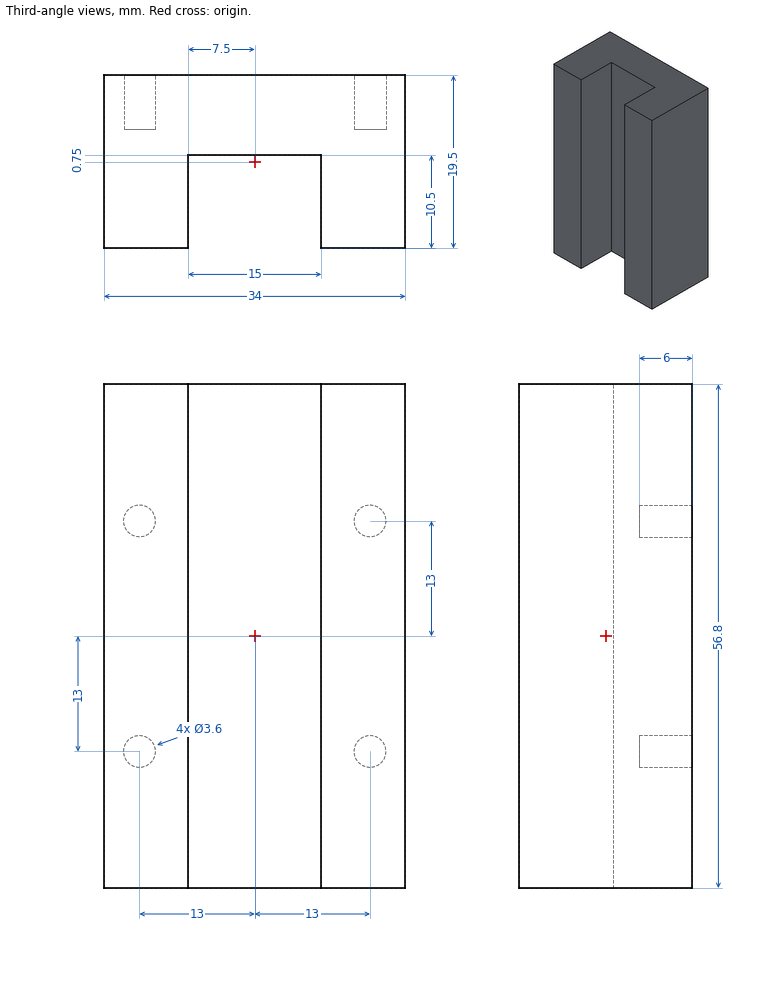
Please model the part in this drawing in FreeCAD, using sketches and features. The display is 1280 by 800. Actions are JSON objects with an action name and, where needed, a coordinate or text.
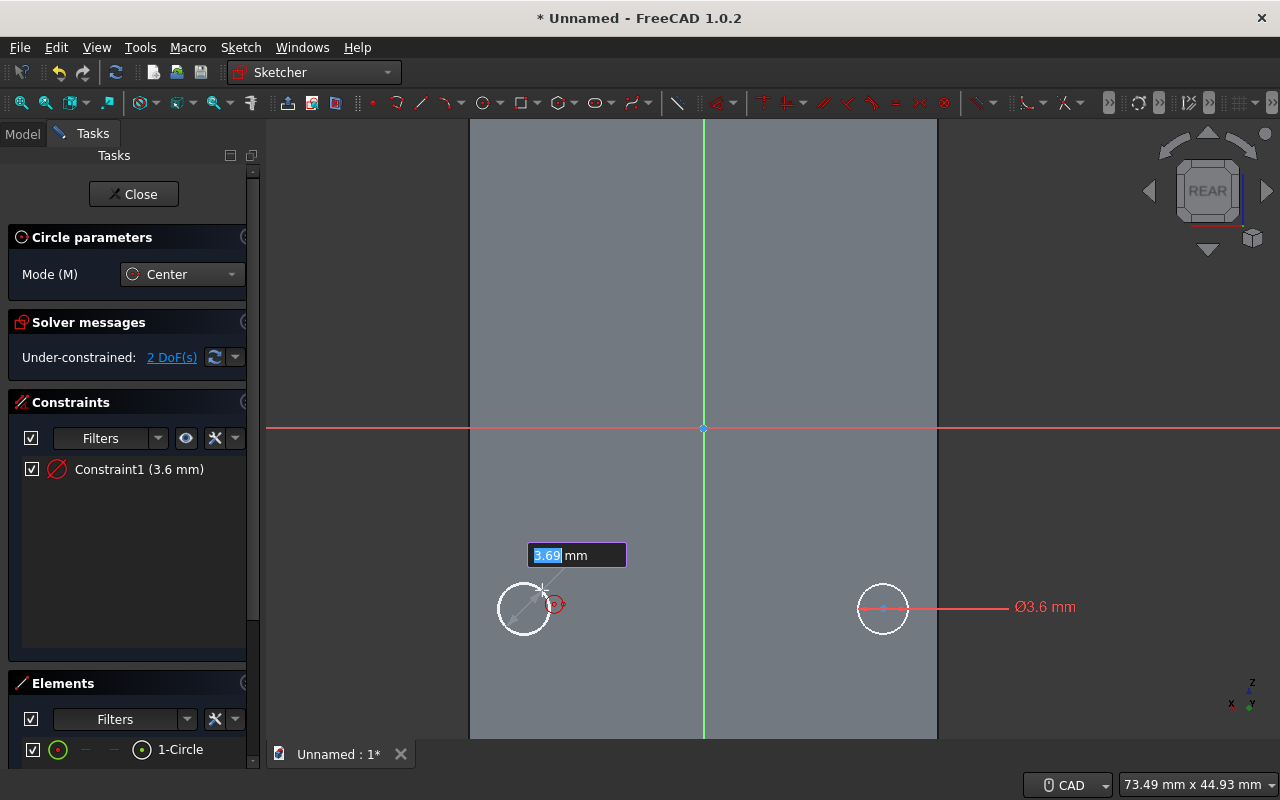
{"action": "type", "text": "3.6"}
{"action": "key", "text": "Return"}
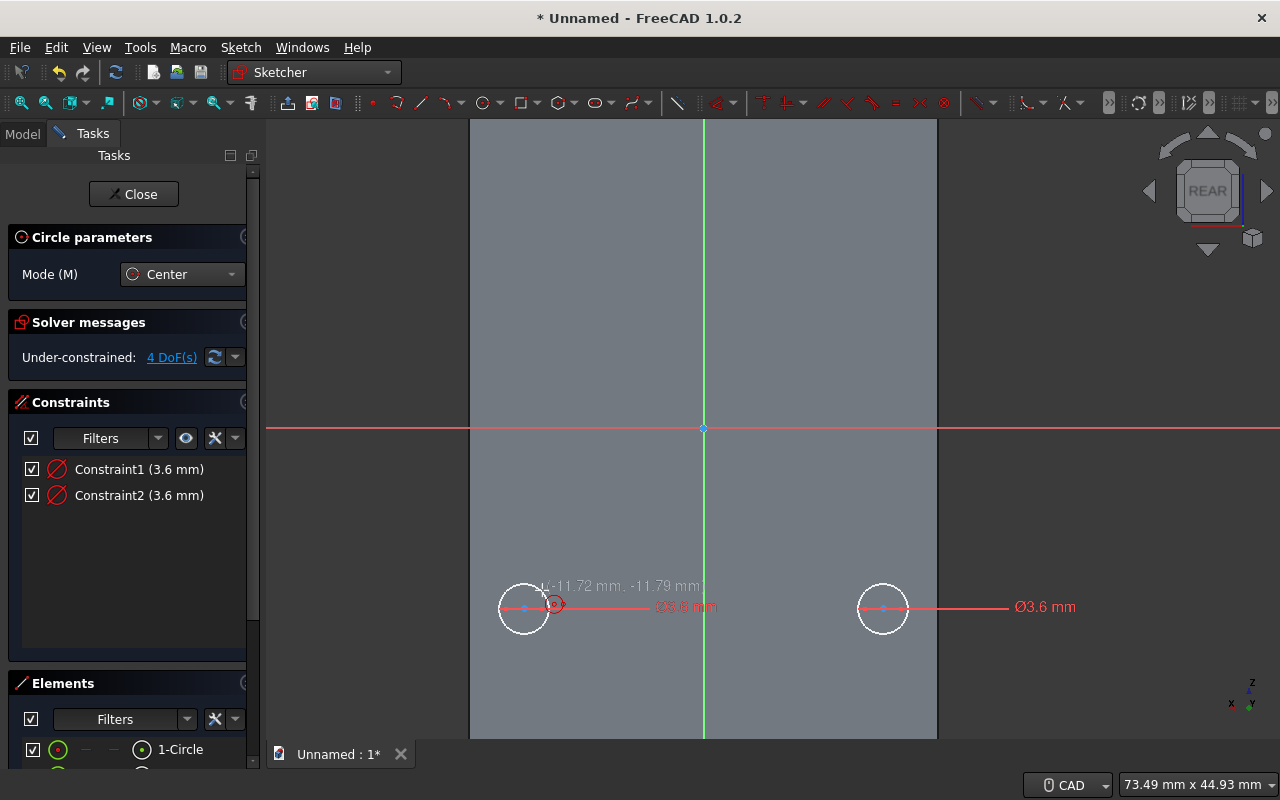
{"action": "left_click", "coordinate": [524, 249]}
{"action": "mouse_move", "coordinate": [542, 231]}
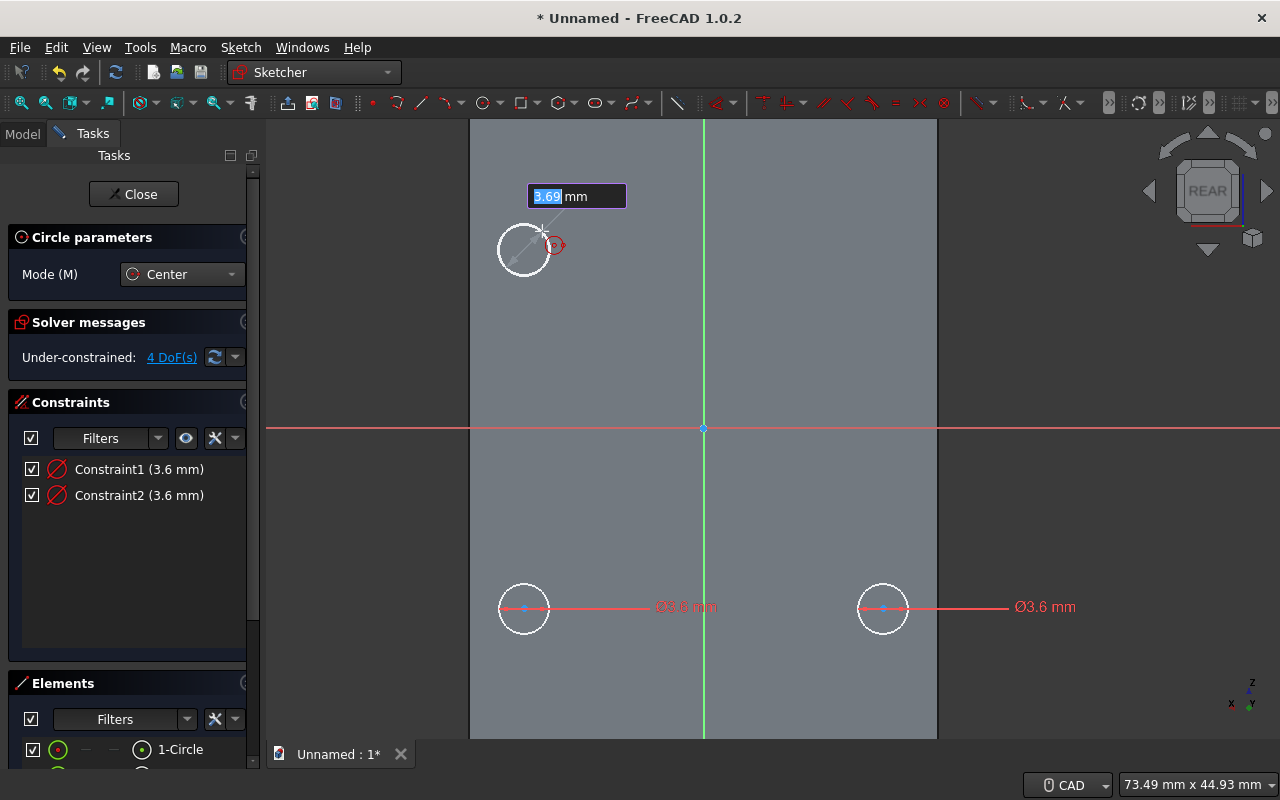
{"action": "type", "text": "3.6"}
{"action": "key", "text": "Return"}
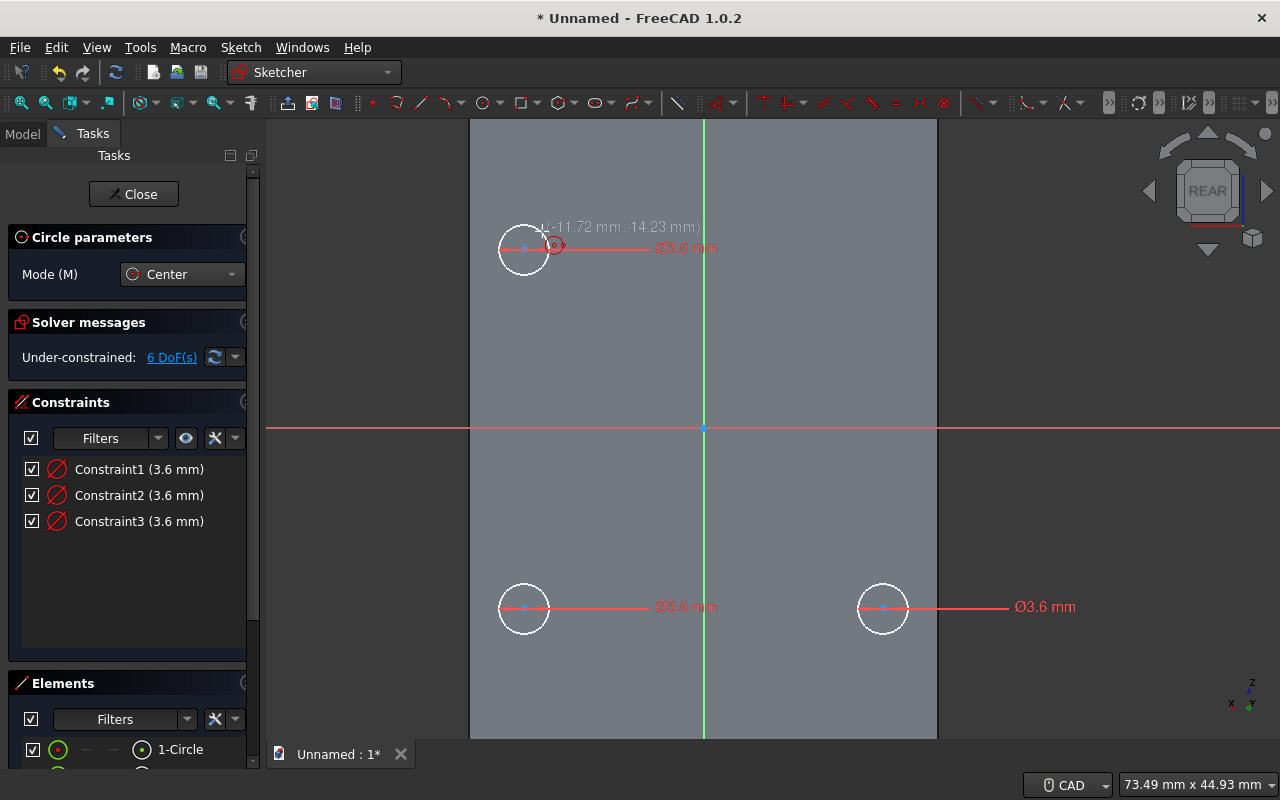
{"action": "left_click", "coordinate": [883, 249]}
{"action": "mouse_move", "coordinate": [901, 231]}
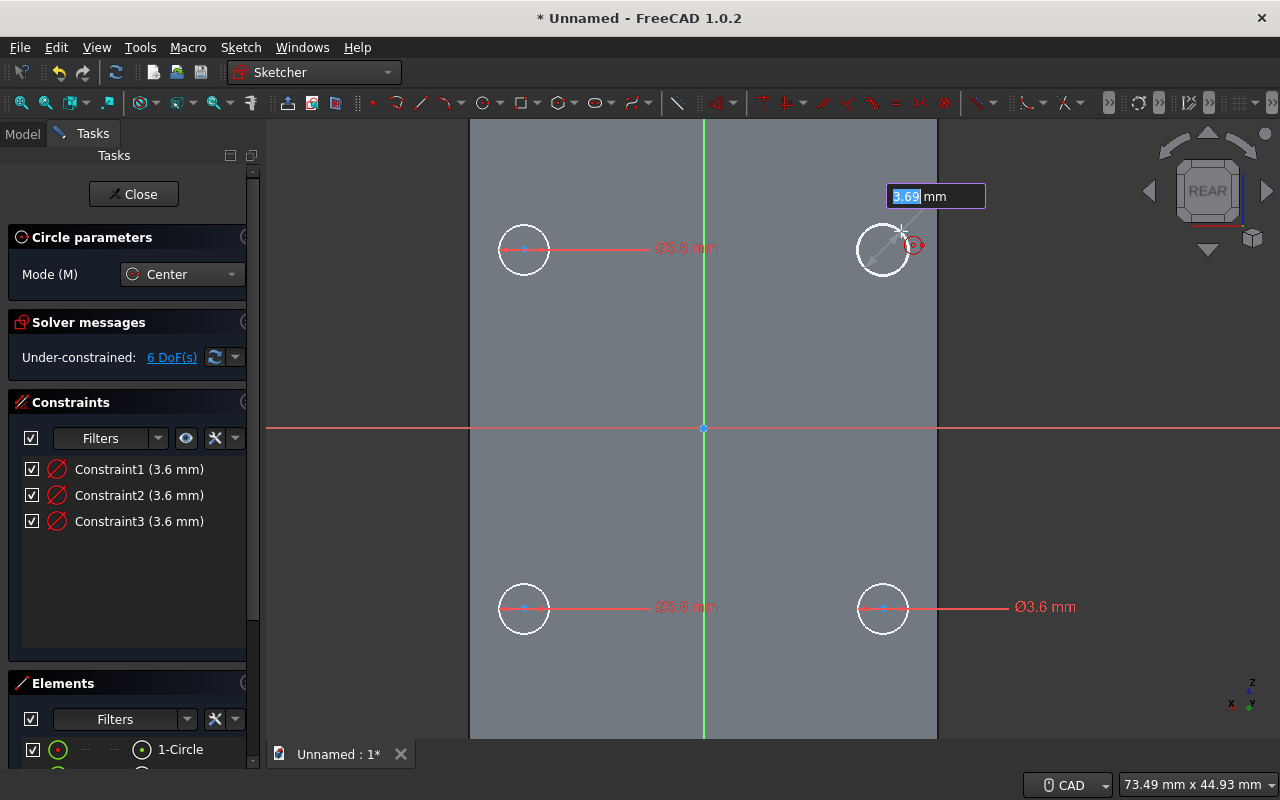
{"action": "type", "text": "3.6"}
{"action": "key", "text": "Return"}
{"action": "key", "text": "Escape"}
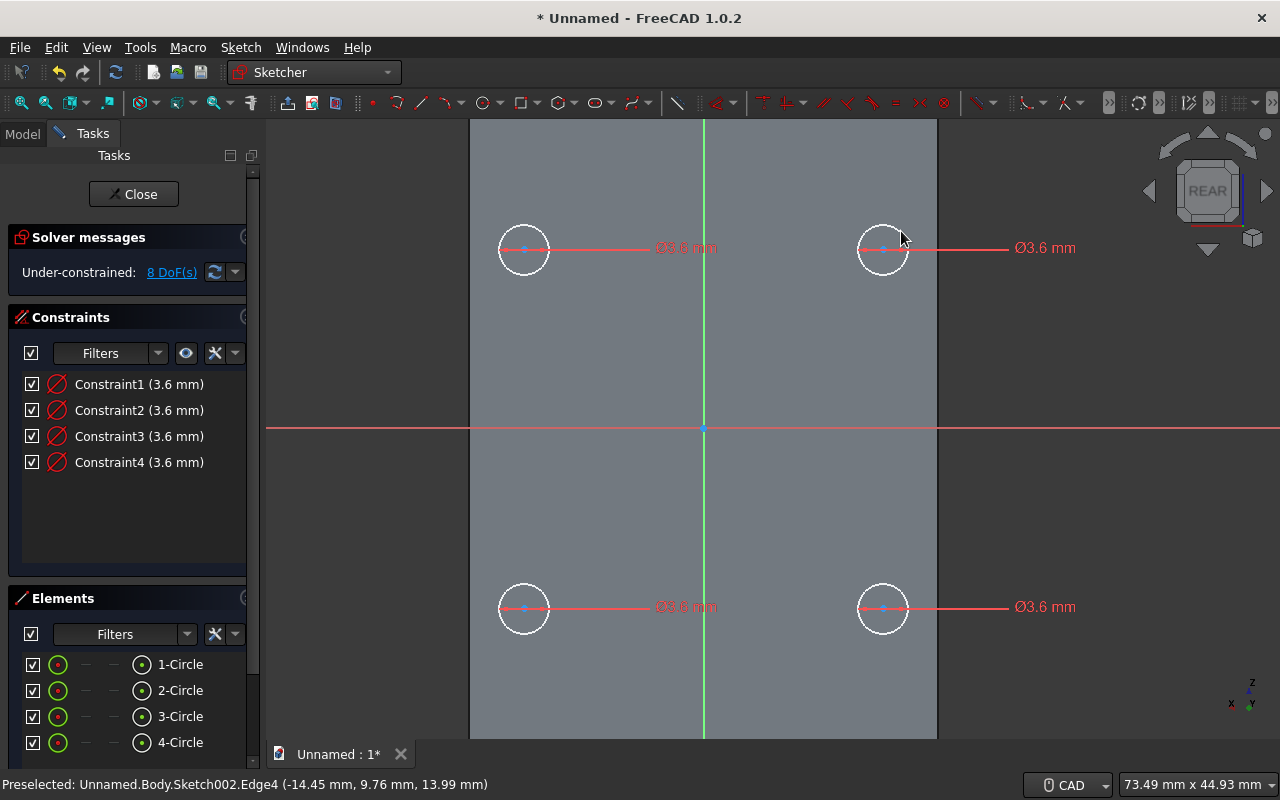
{"action": "left_click", "coordinate": [883, 609]}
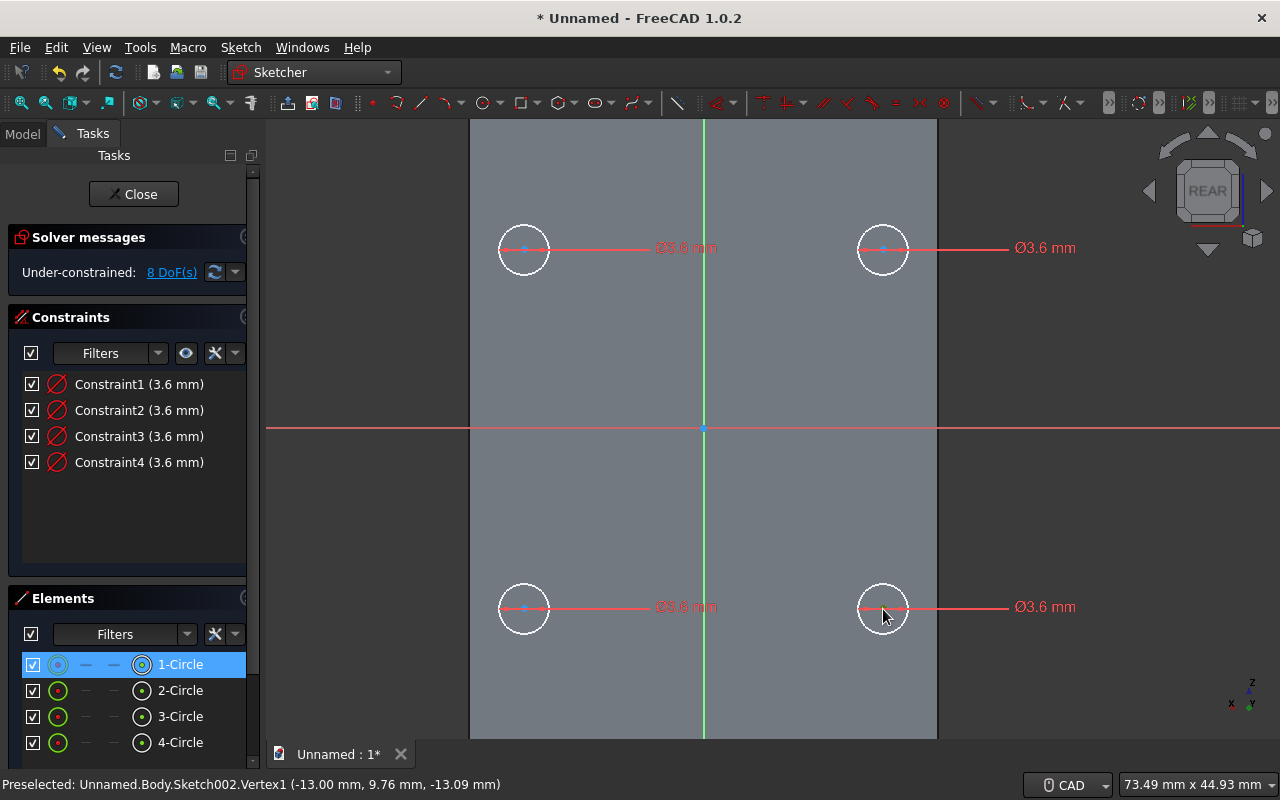
{"action": "left_click", "coordinate": [524, 609]}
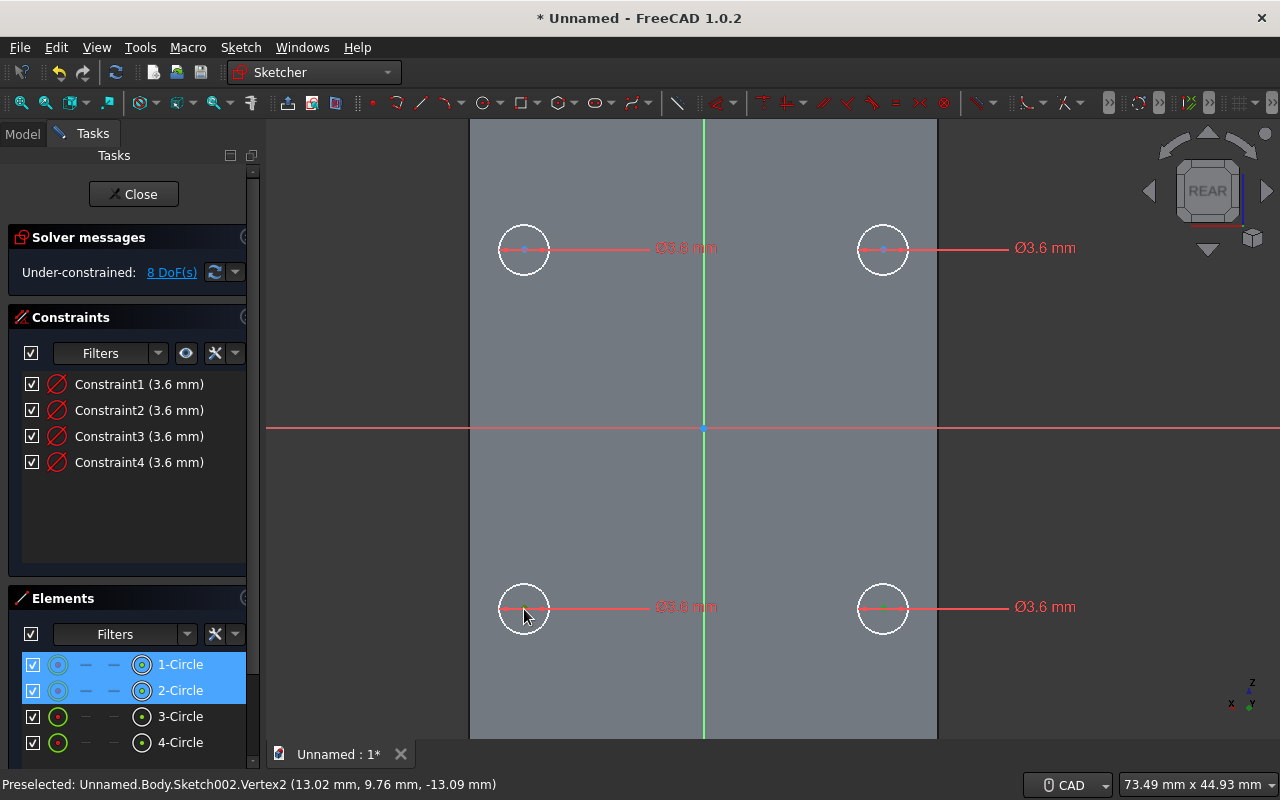
{"action": "key", "text": "h"}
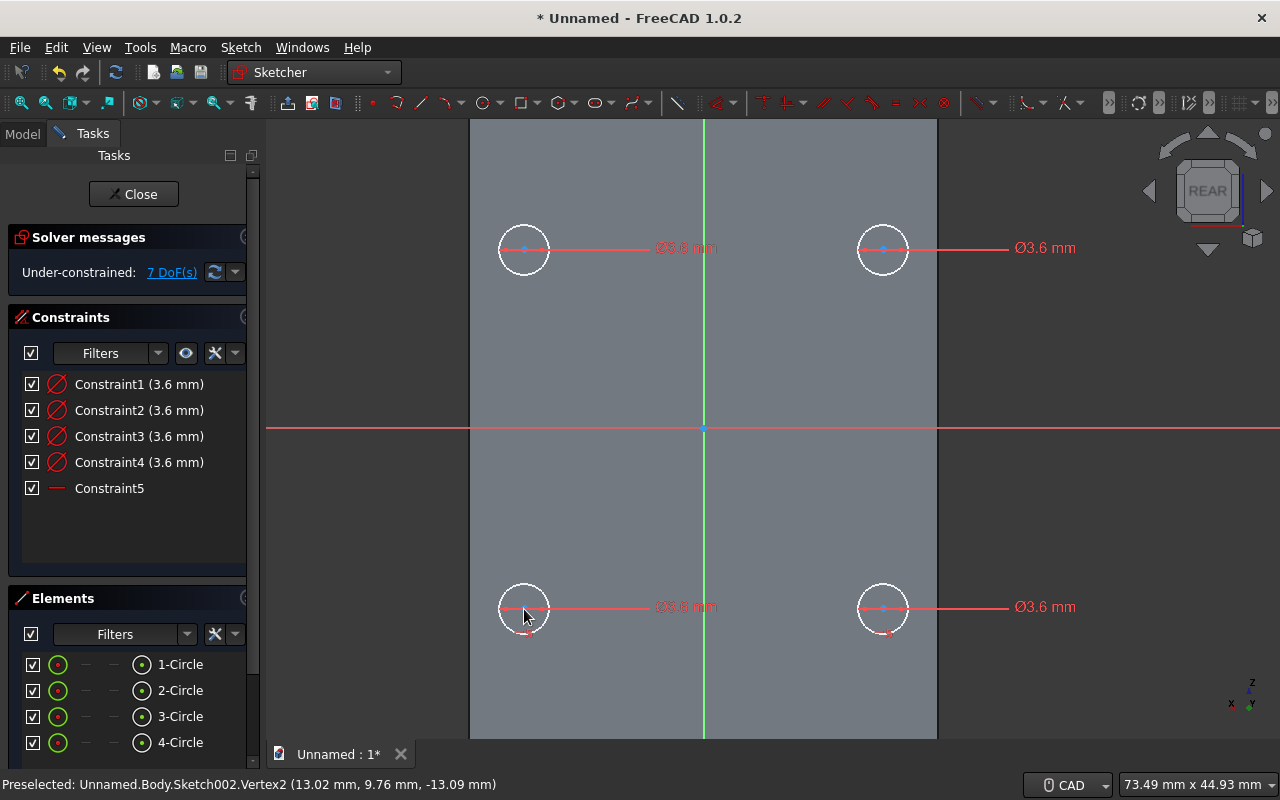
{"action": "left_click", "coordinate": [524, 609]}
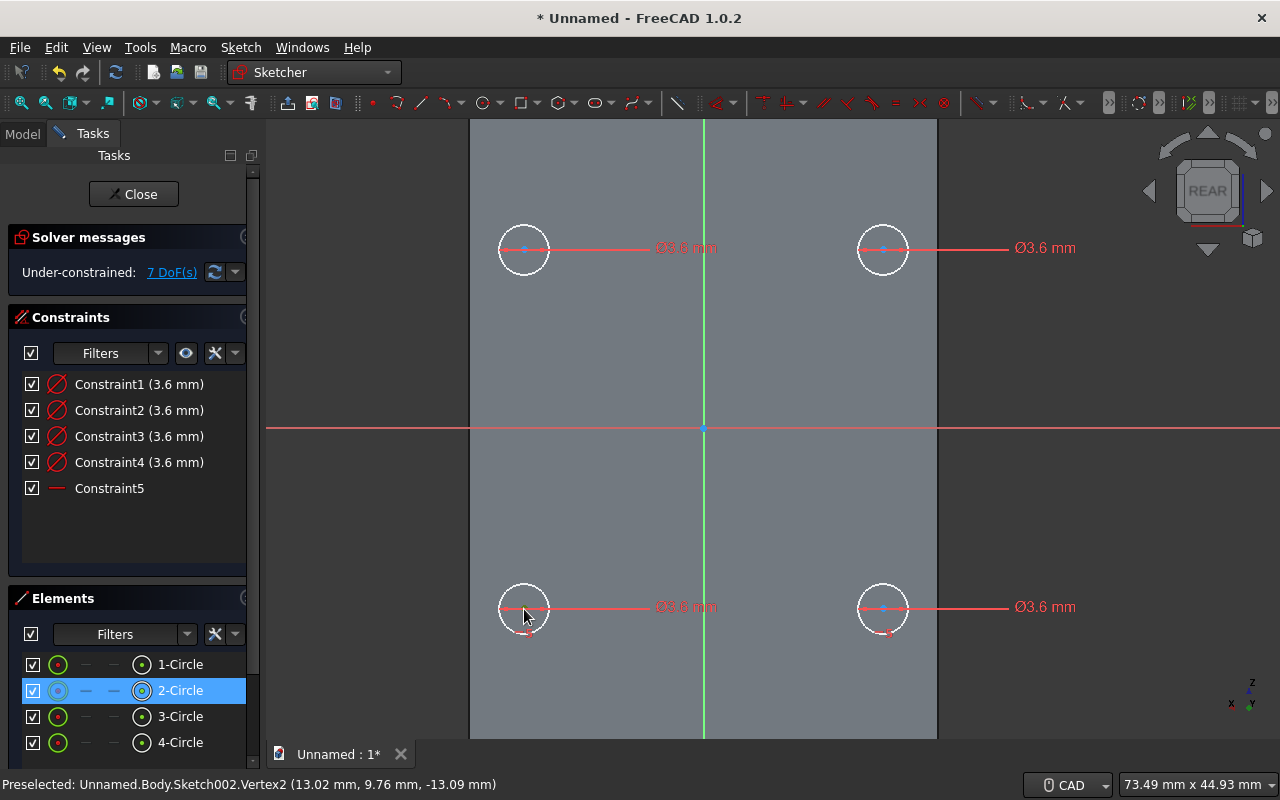
{"action": "left_click", "coordinate": [524, 250]}